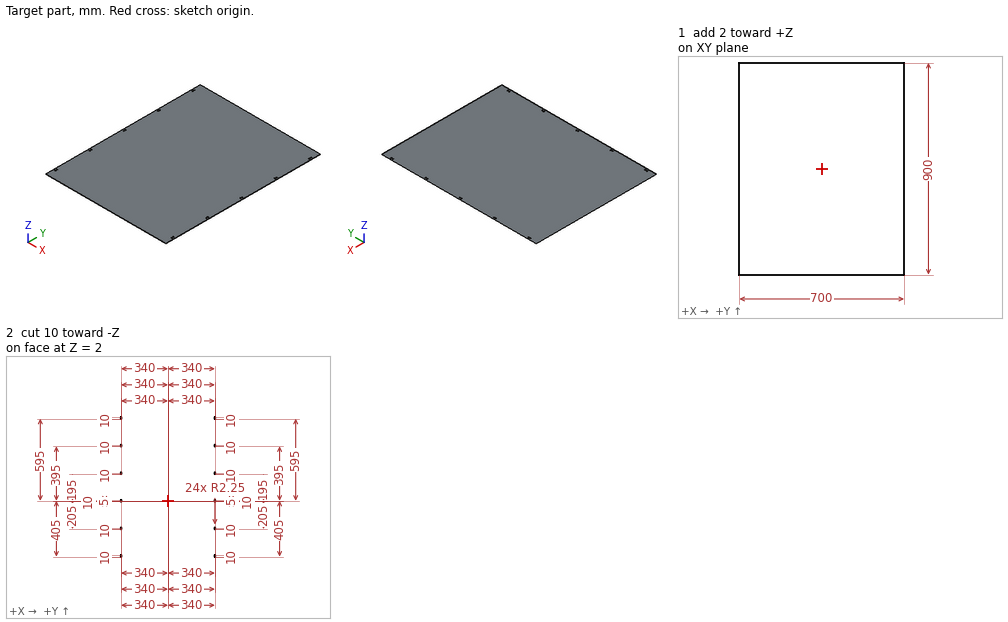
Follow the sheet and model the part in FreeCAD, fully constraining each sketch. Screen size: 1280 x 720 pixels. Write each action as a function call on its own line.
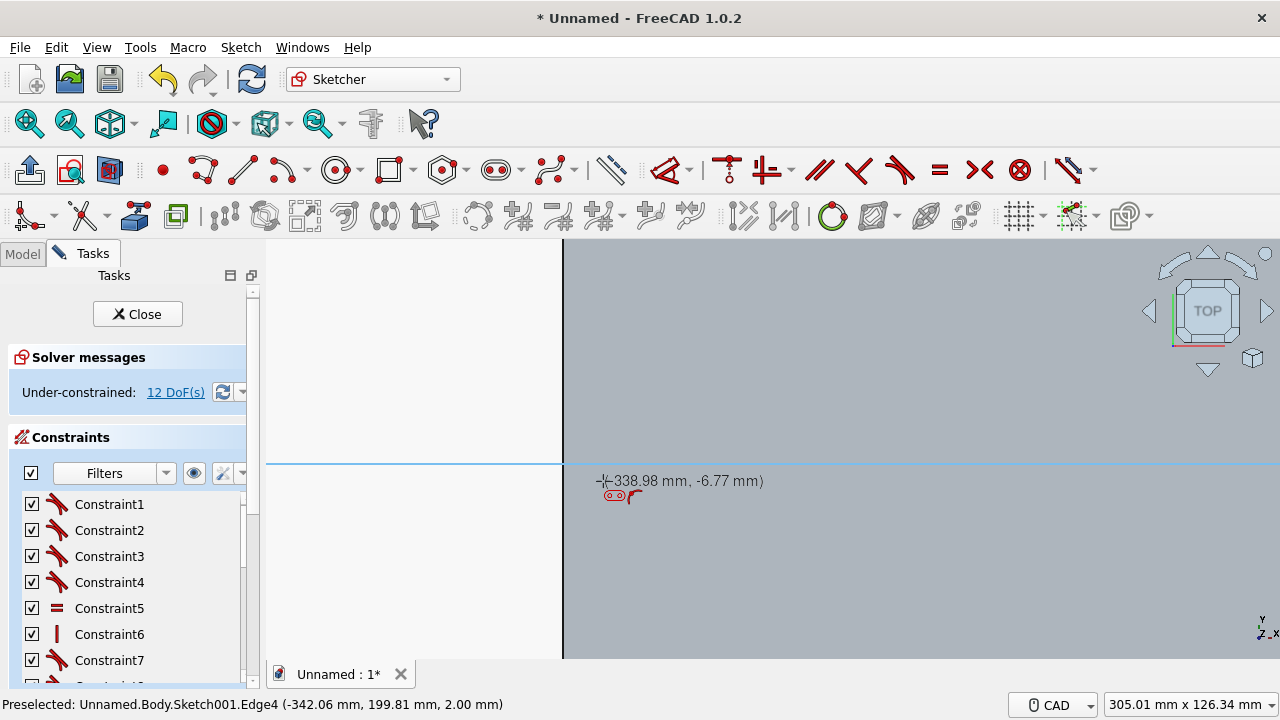
click(596, 480)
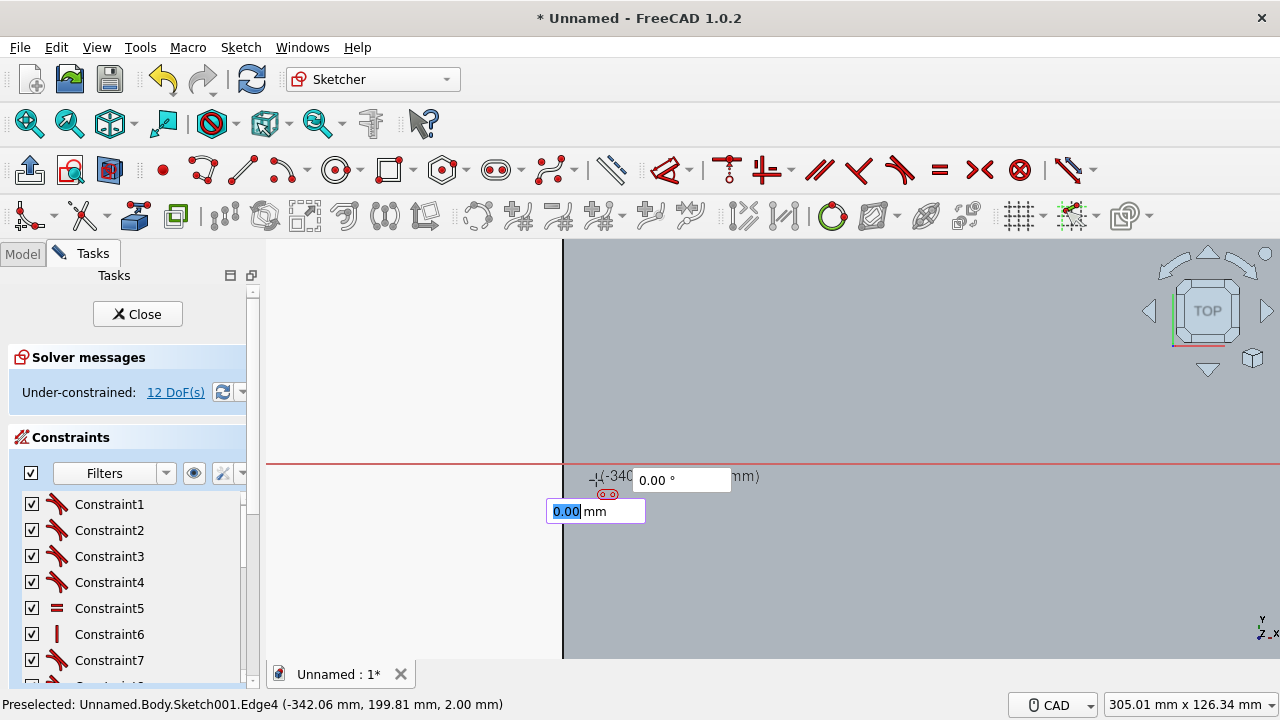
click(596, 447)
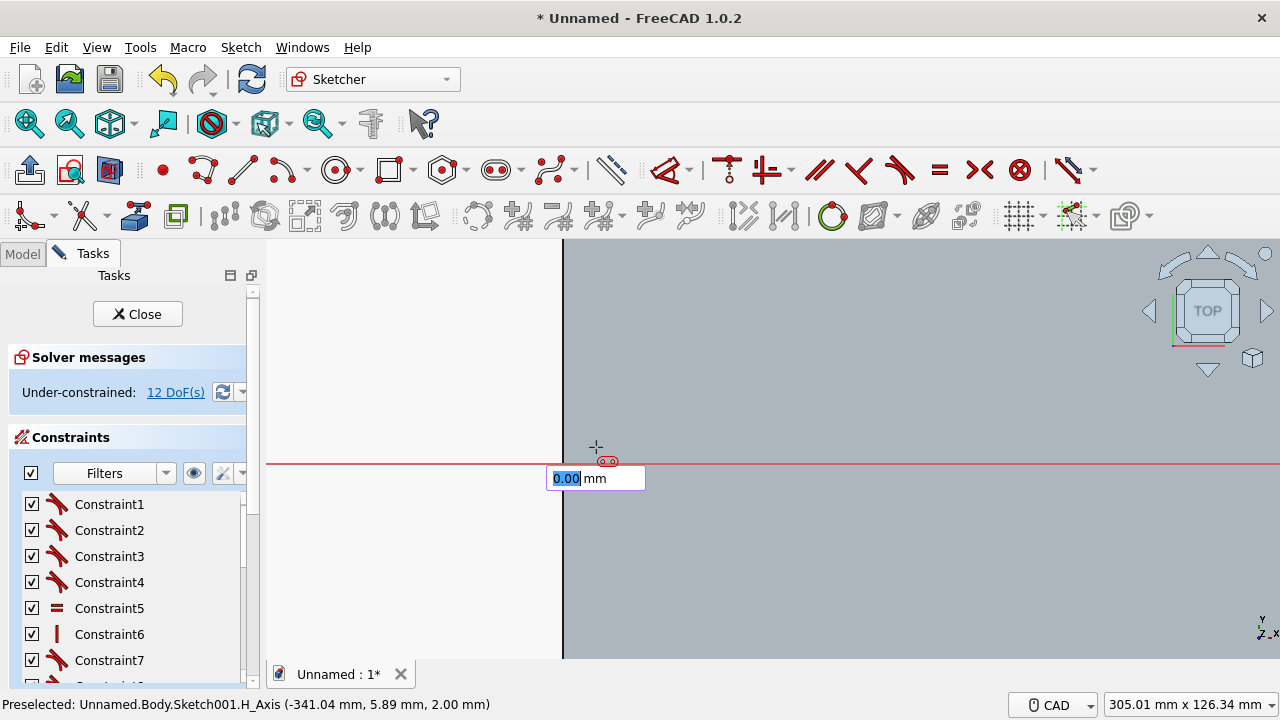
scroll(589, 459, up, 6)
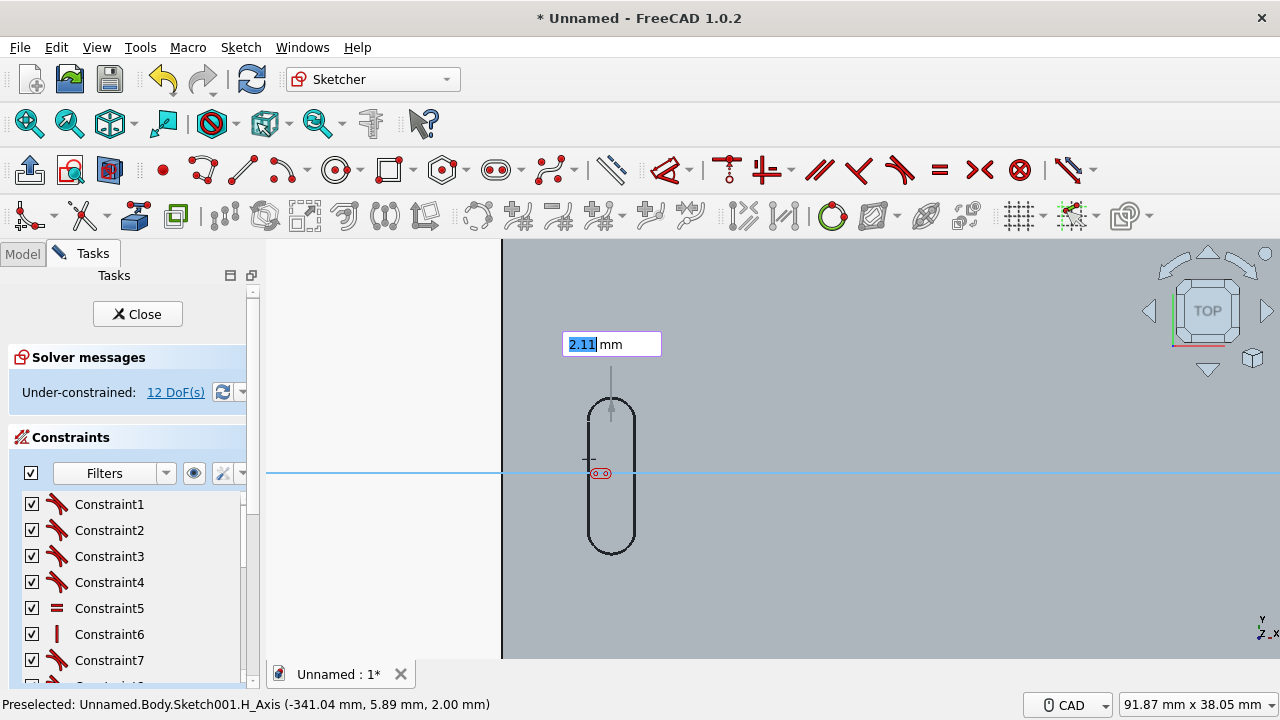
click(588, 457)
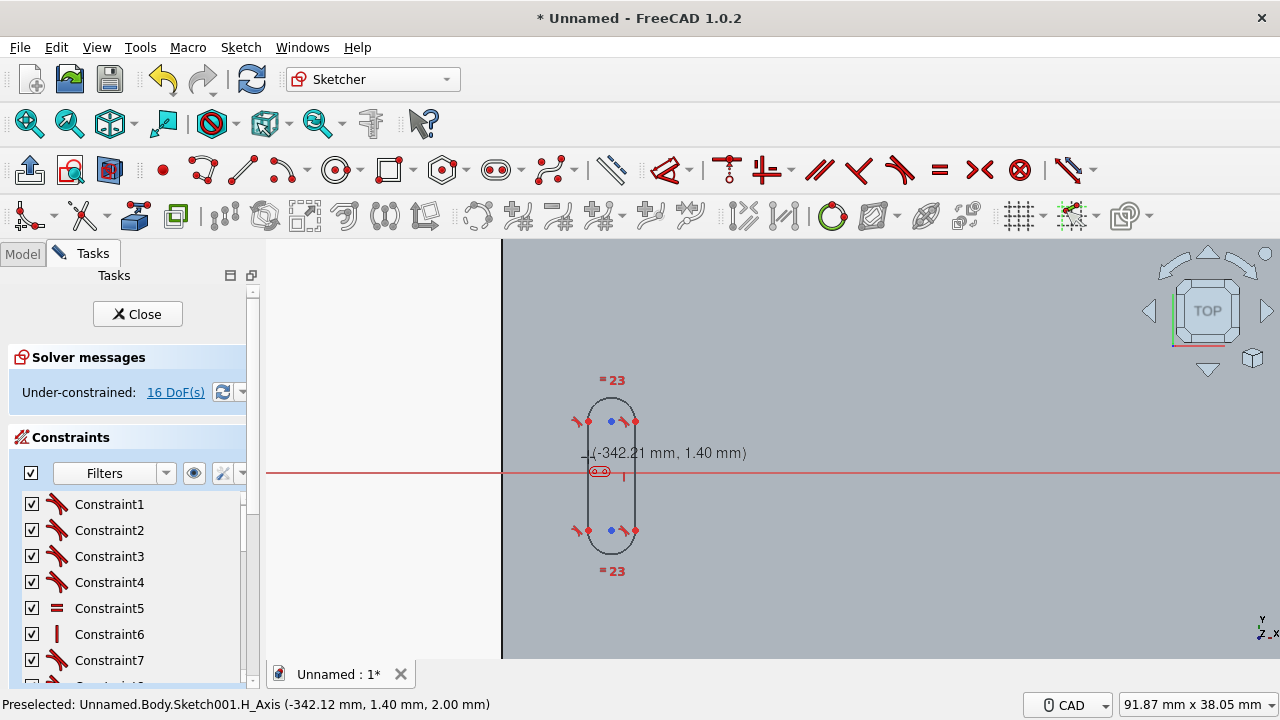
scroll(602, 479, down, 18)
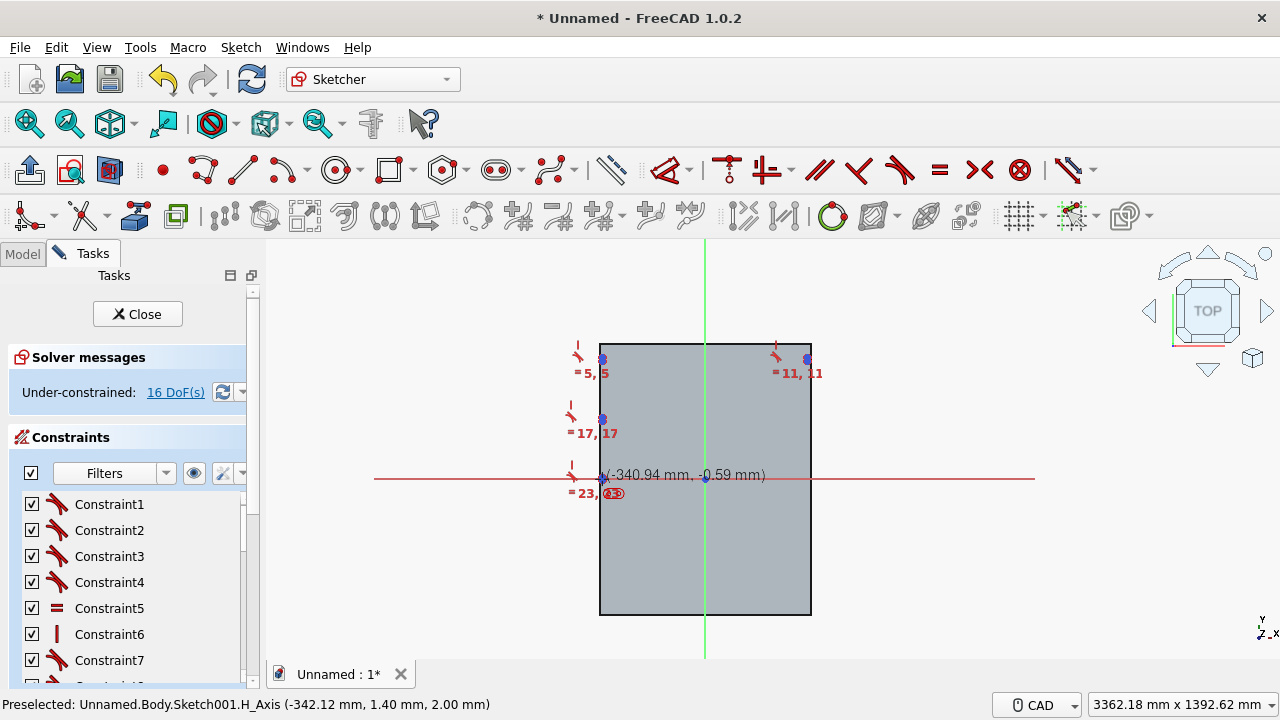
scroll(808, 421, up, 18)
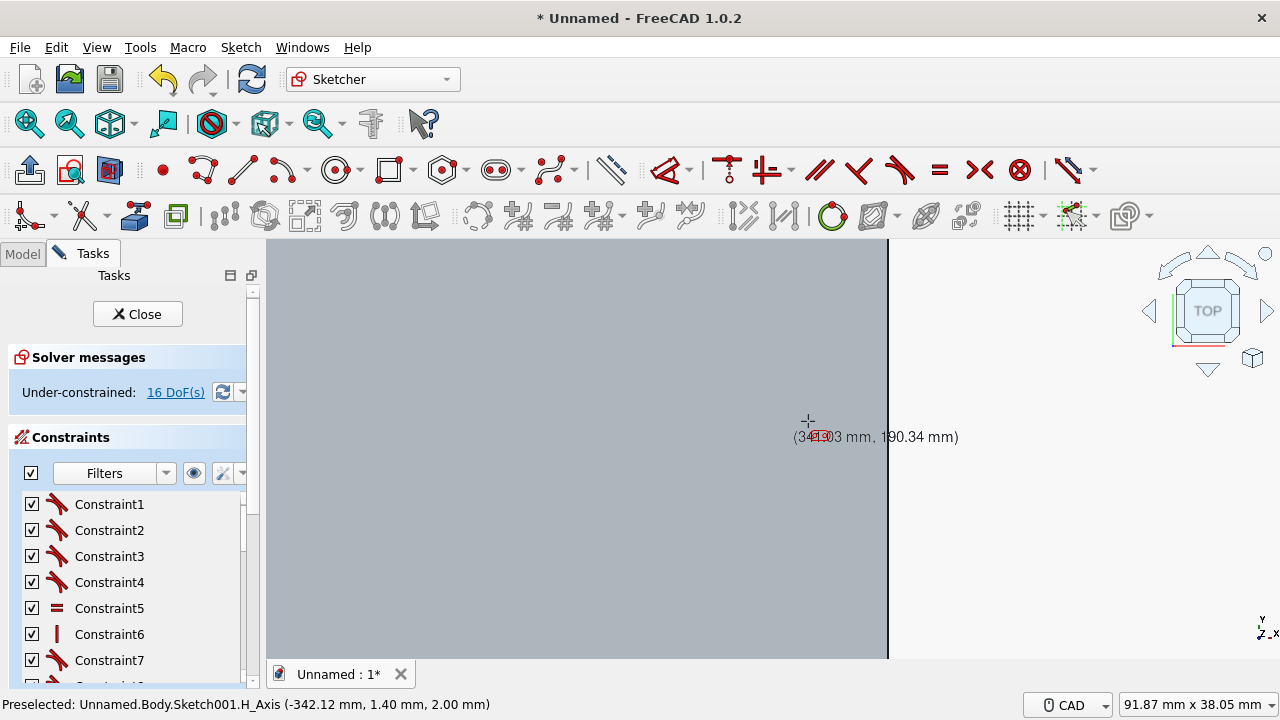
scroll(808, 421, down, 18)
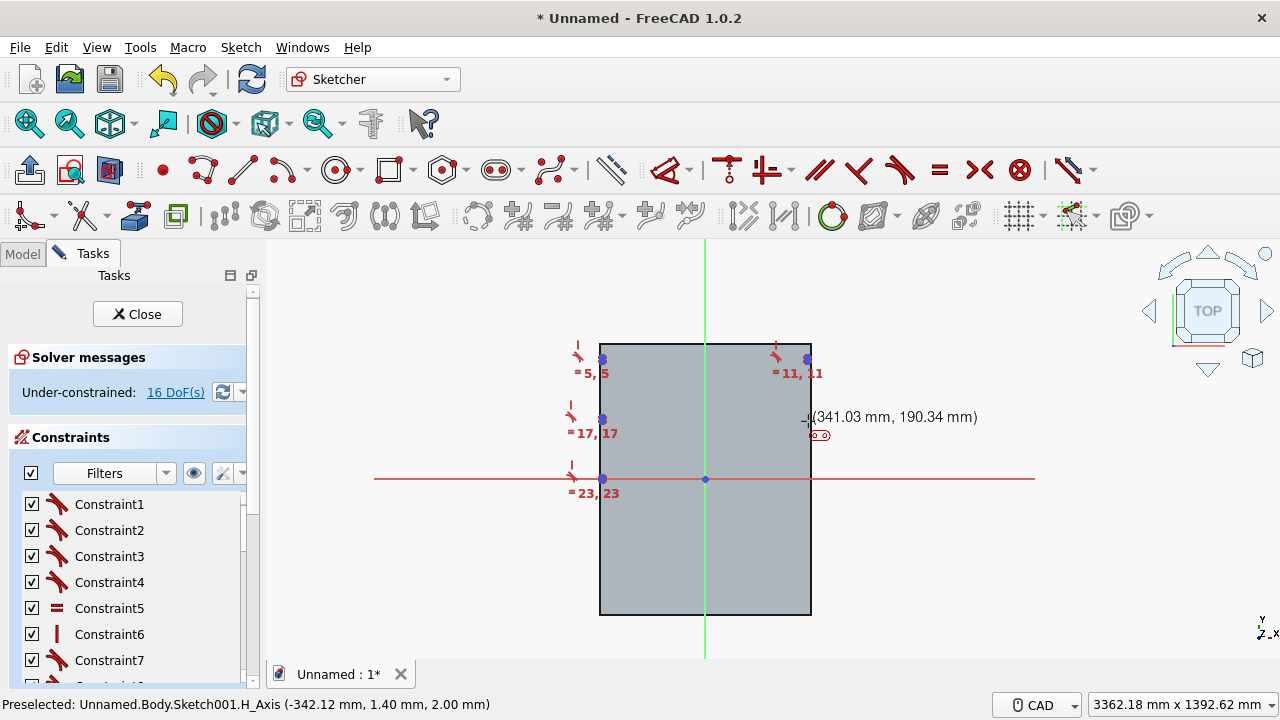
click(808, 421)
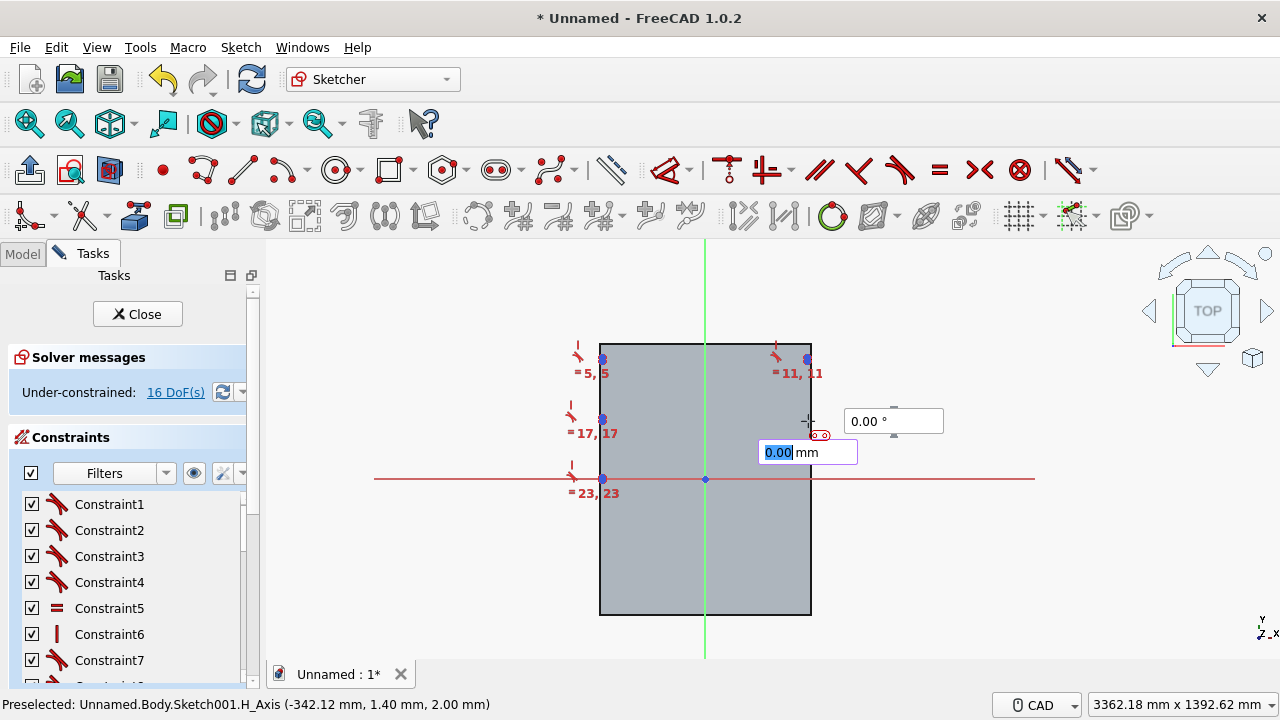
scroll(808, 418, up, 9)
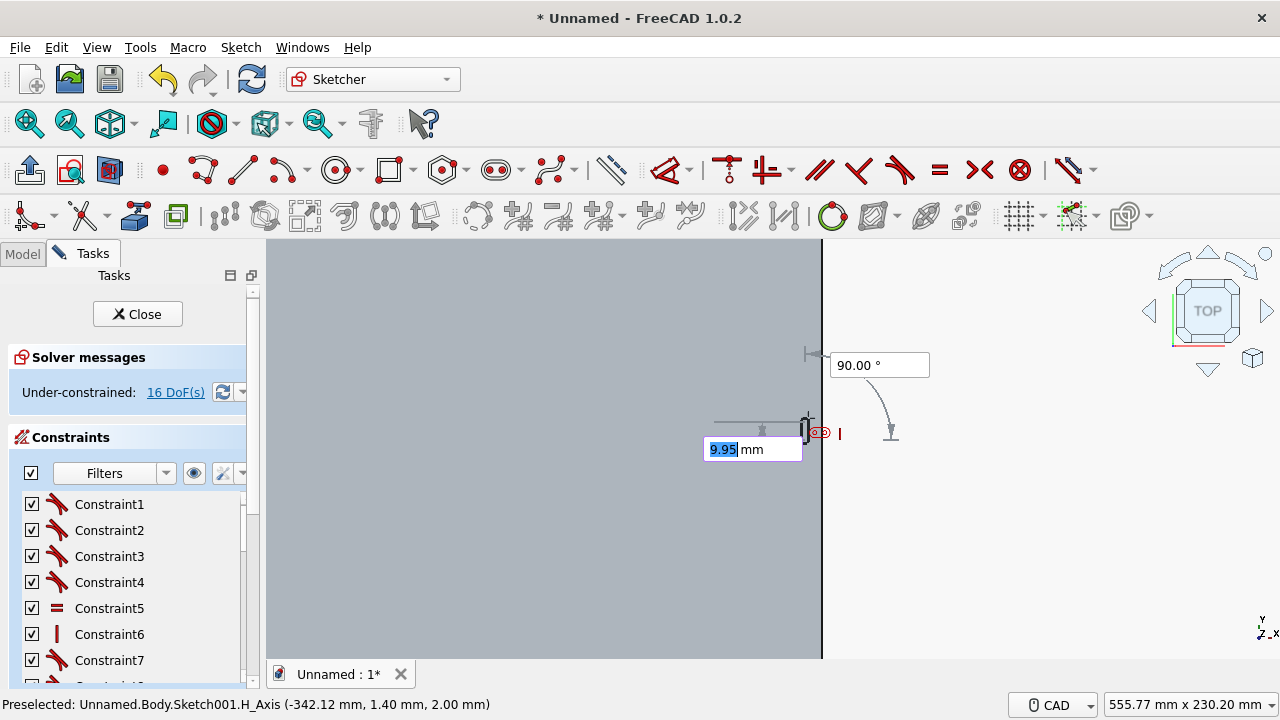
click(805, 413)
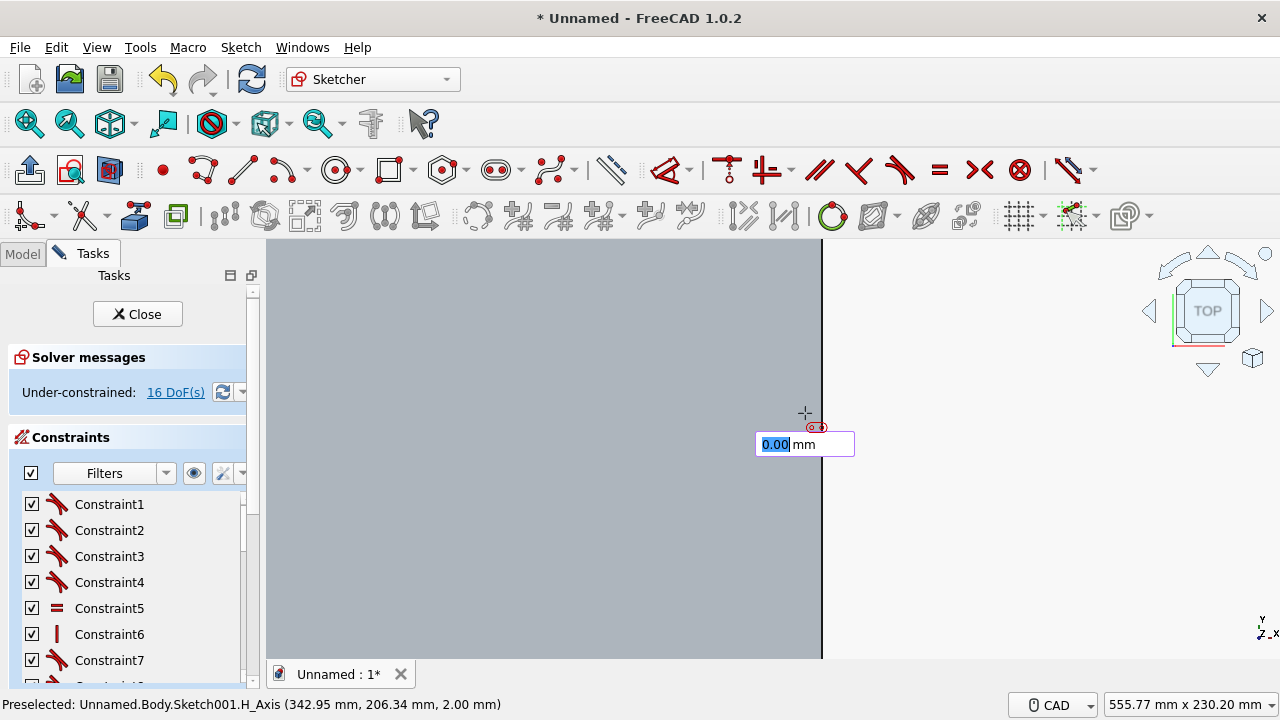
scroll(808, 422, up, 7)